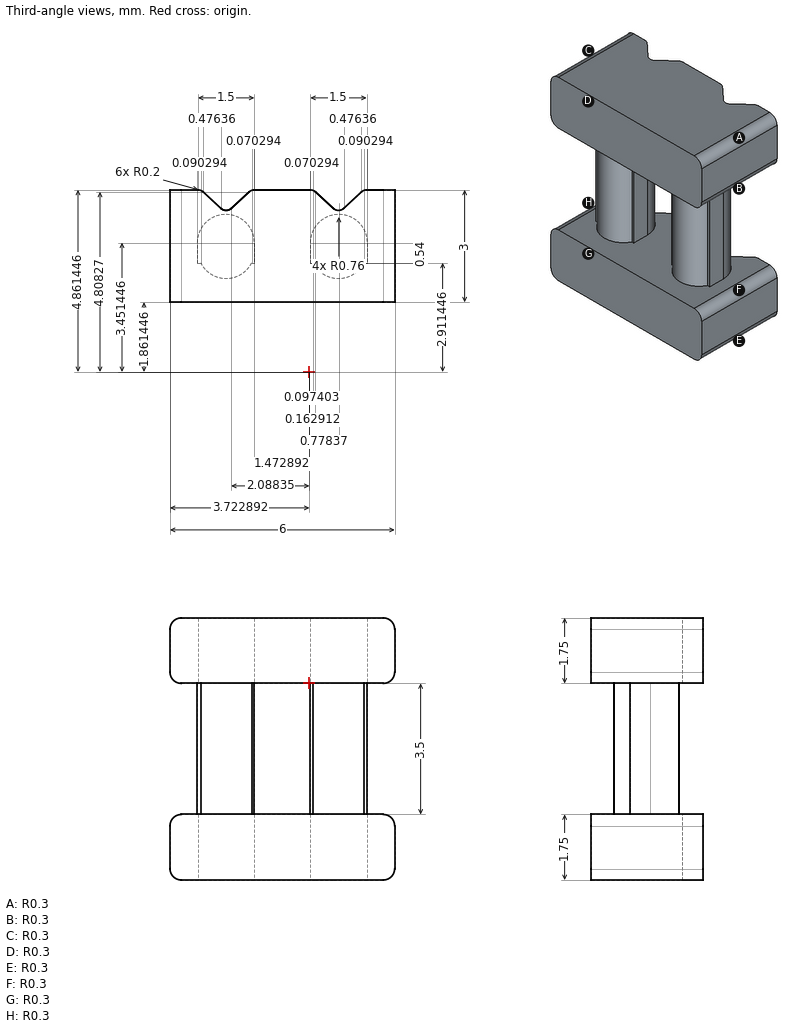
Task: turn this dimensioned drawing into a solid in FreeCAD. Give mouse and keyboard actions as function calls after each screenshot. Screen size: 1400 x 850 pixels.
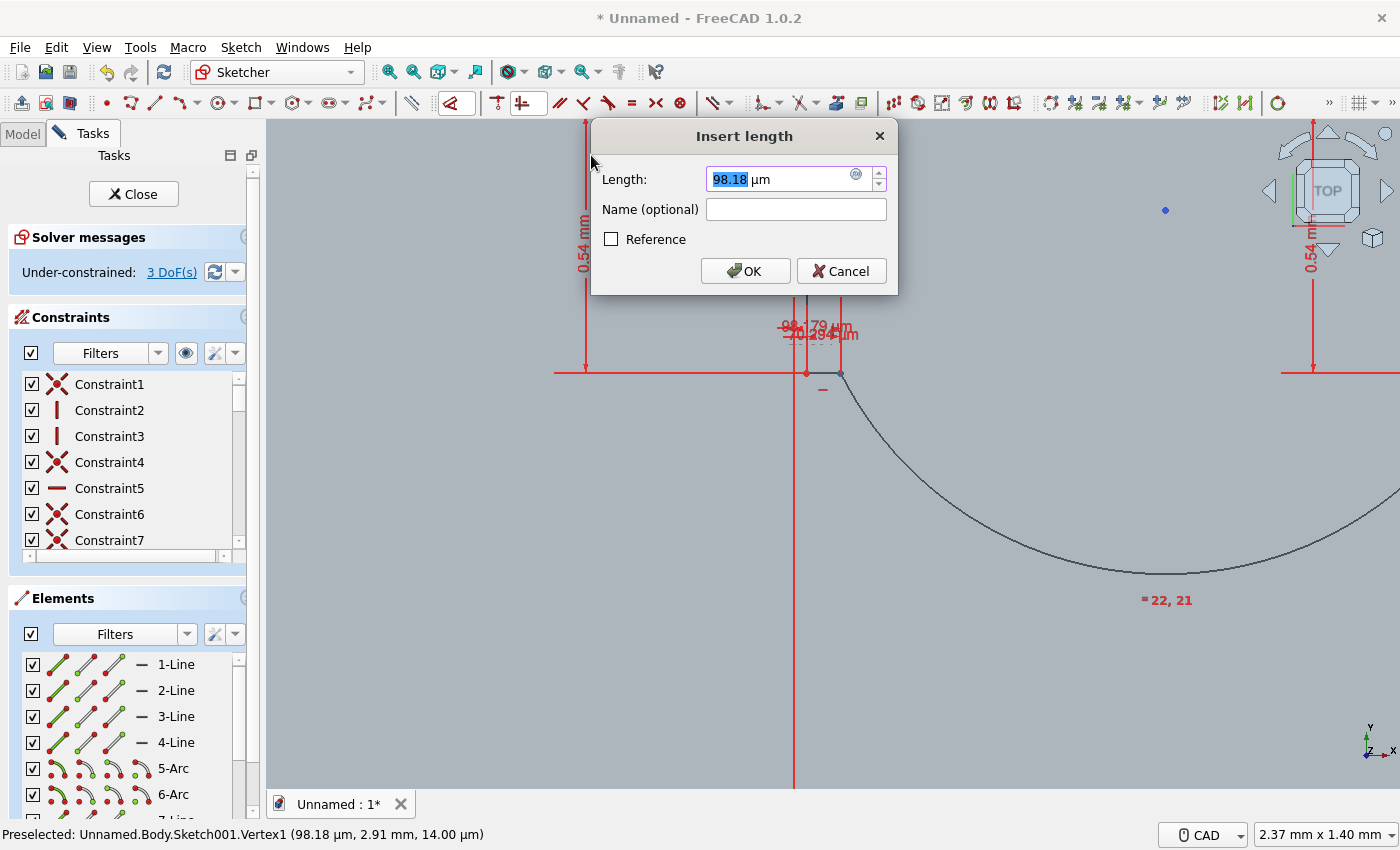
key(ctrl+a)
text(0.097403 mm)
key(Return)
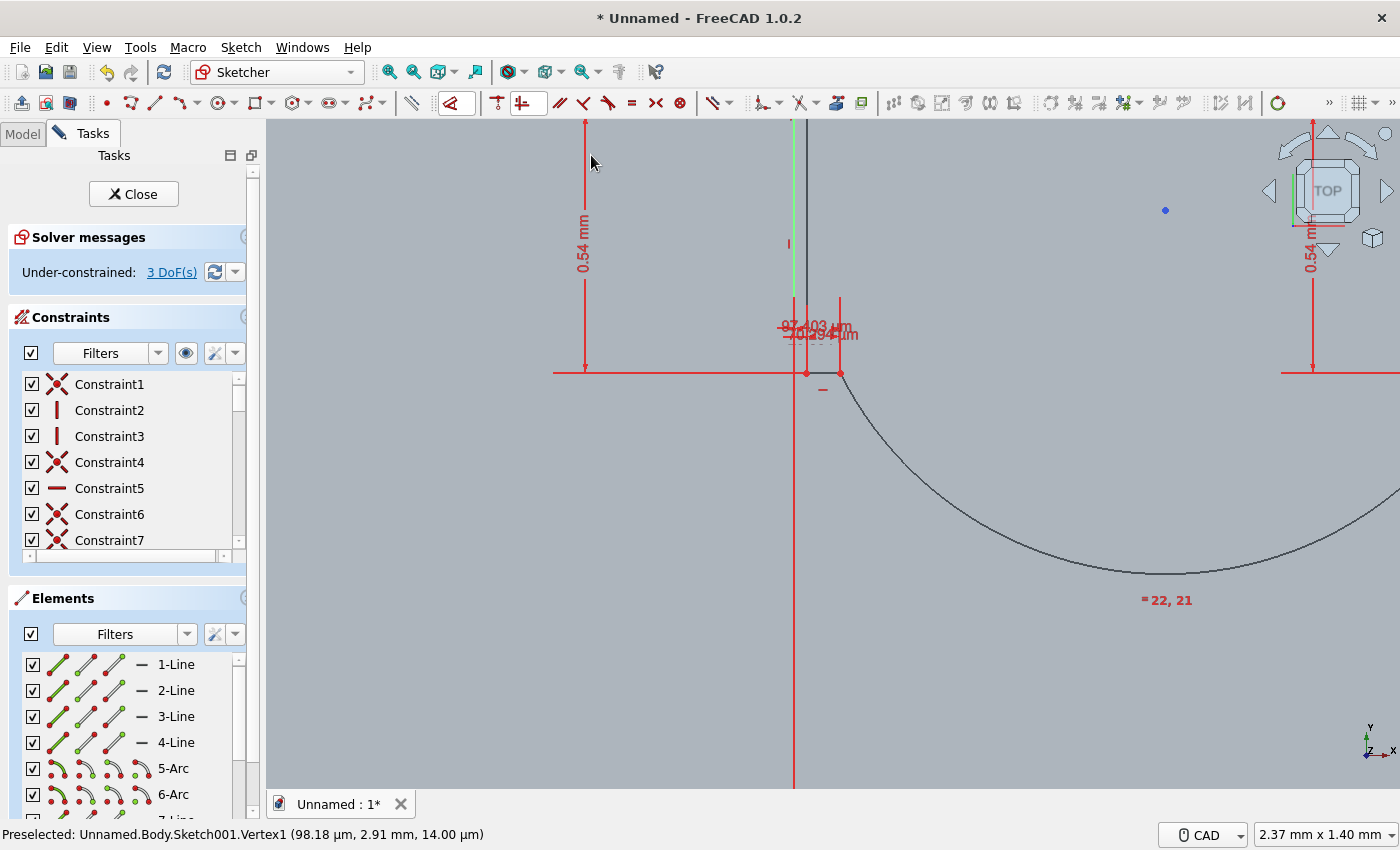
click(840, 373)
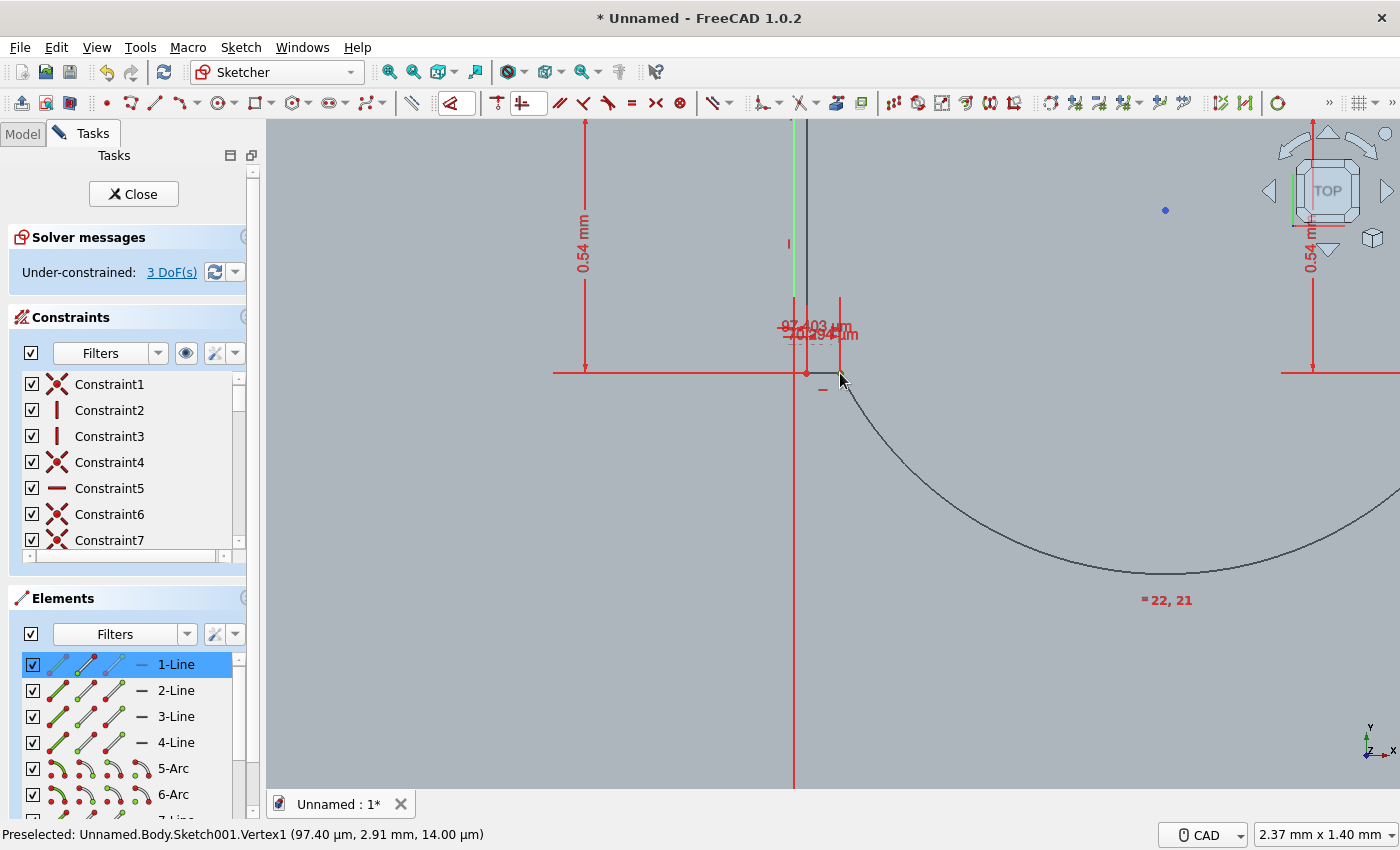
key(i)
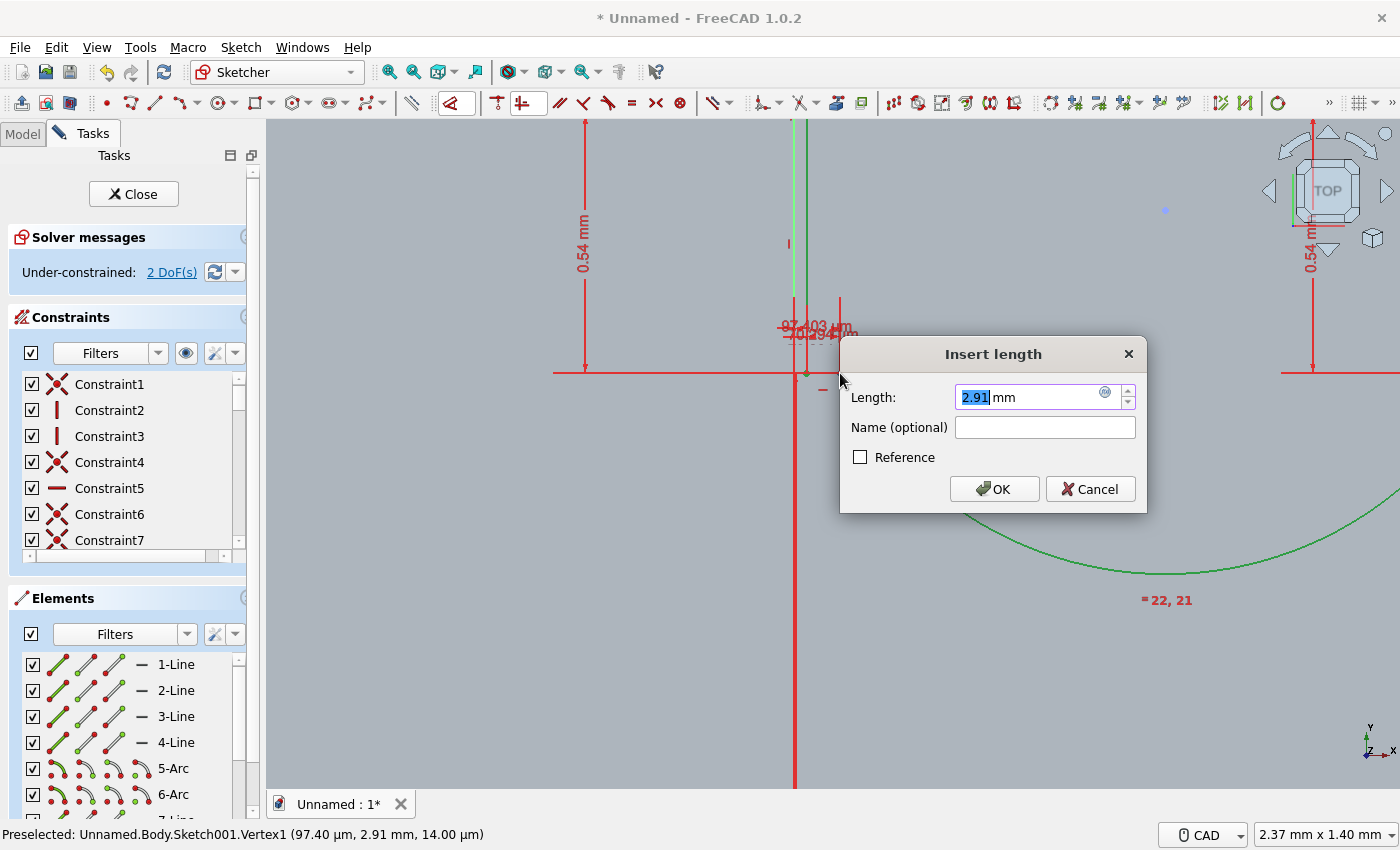
text(2.911446)
key(Return)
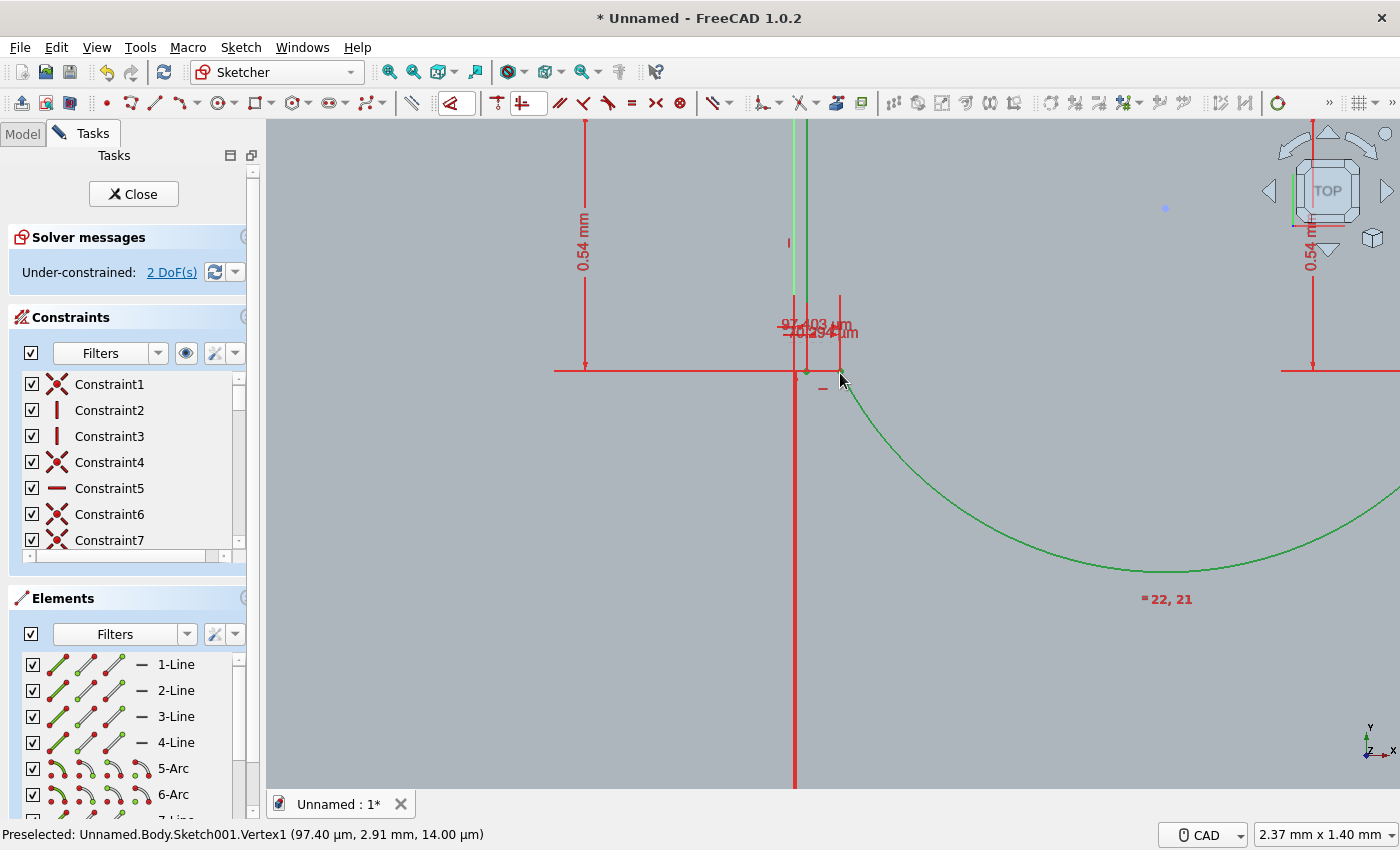
scroll(845, 377, down, 8)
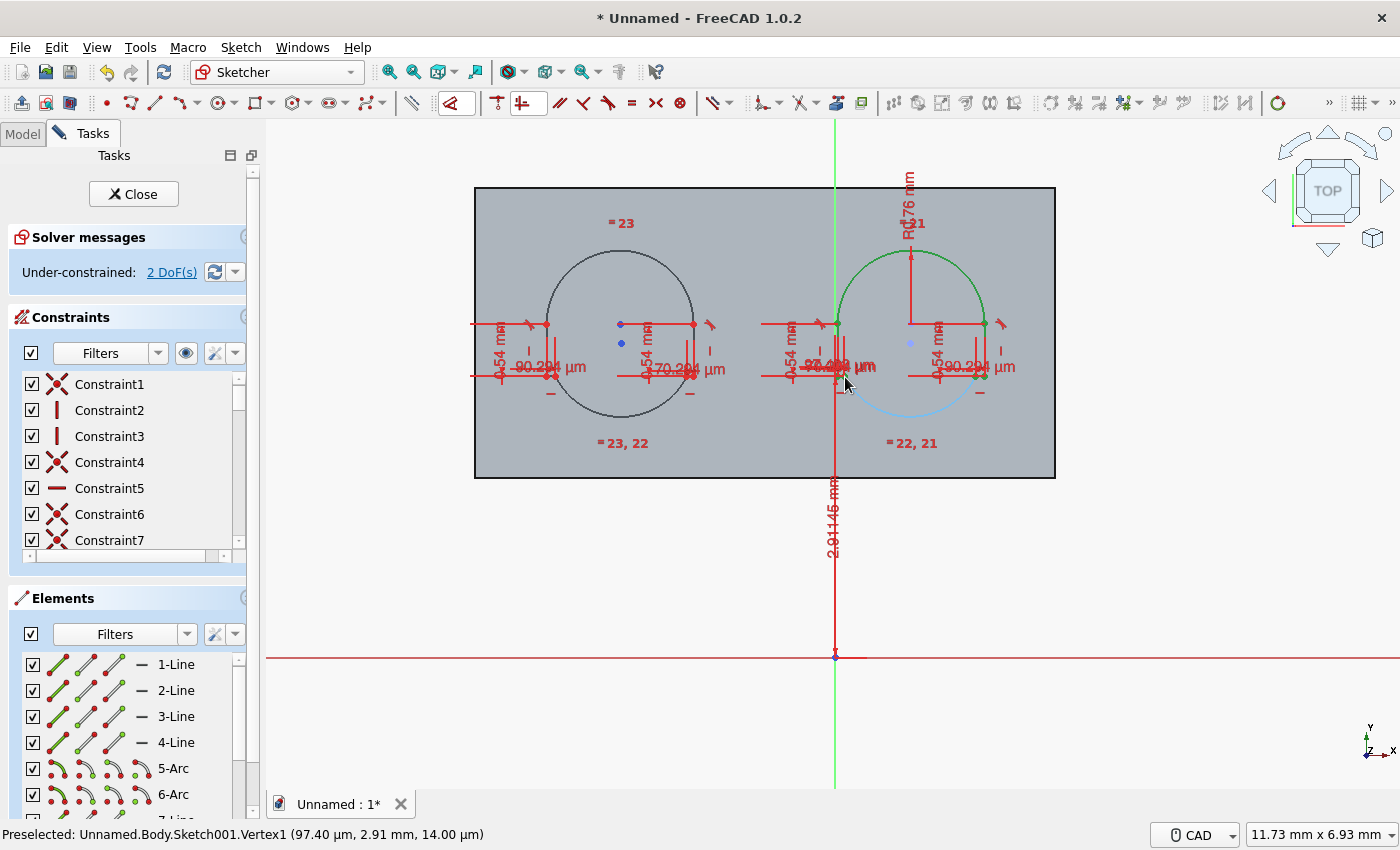
click(694, 324)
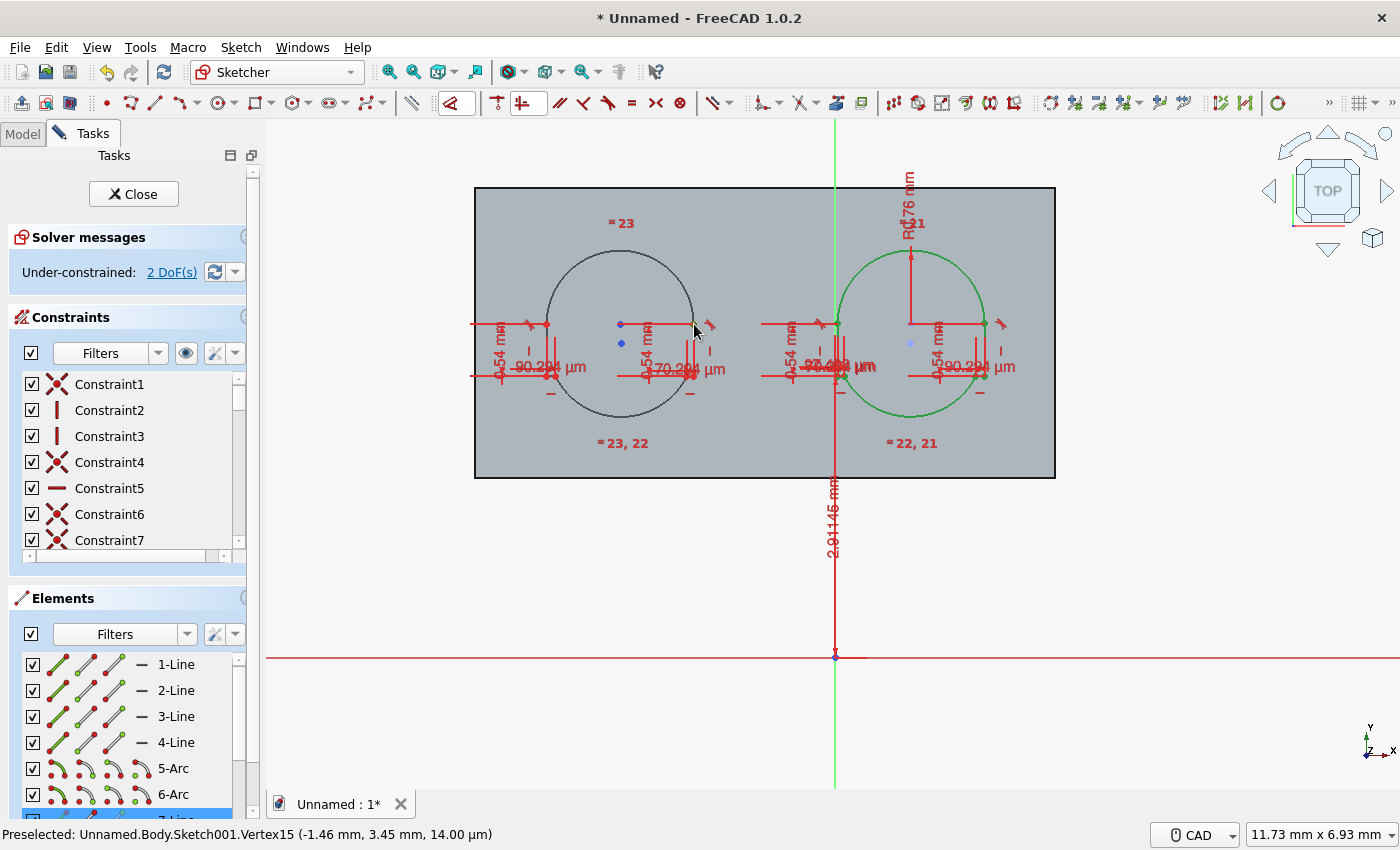
key(l)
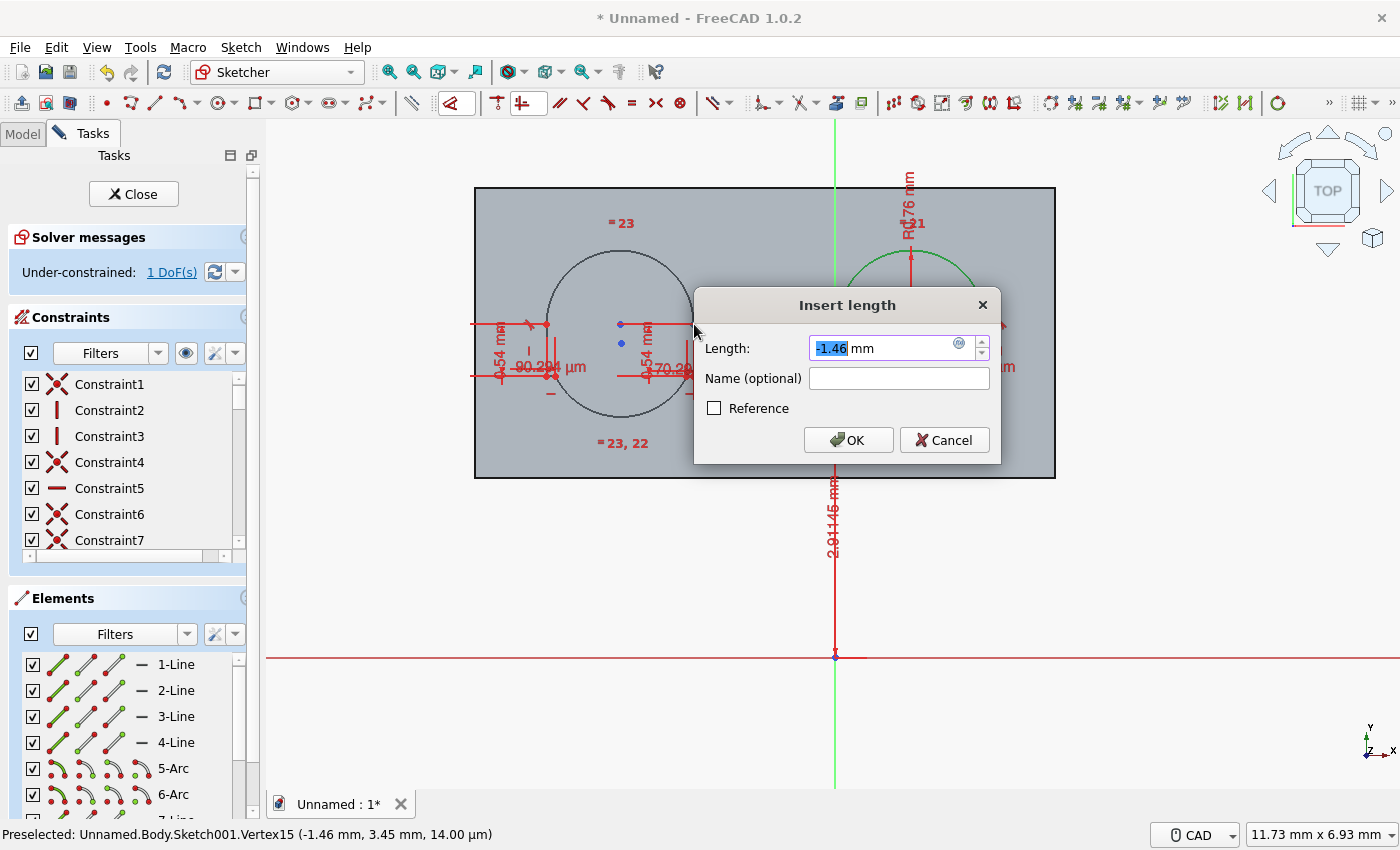
text(-1.472892)
key(Return)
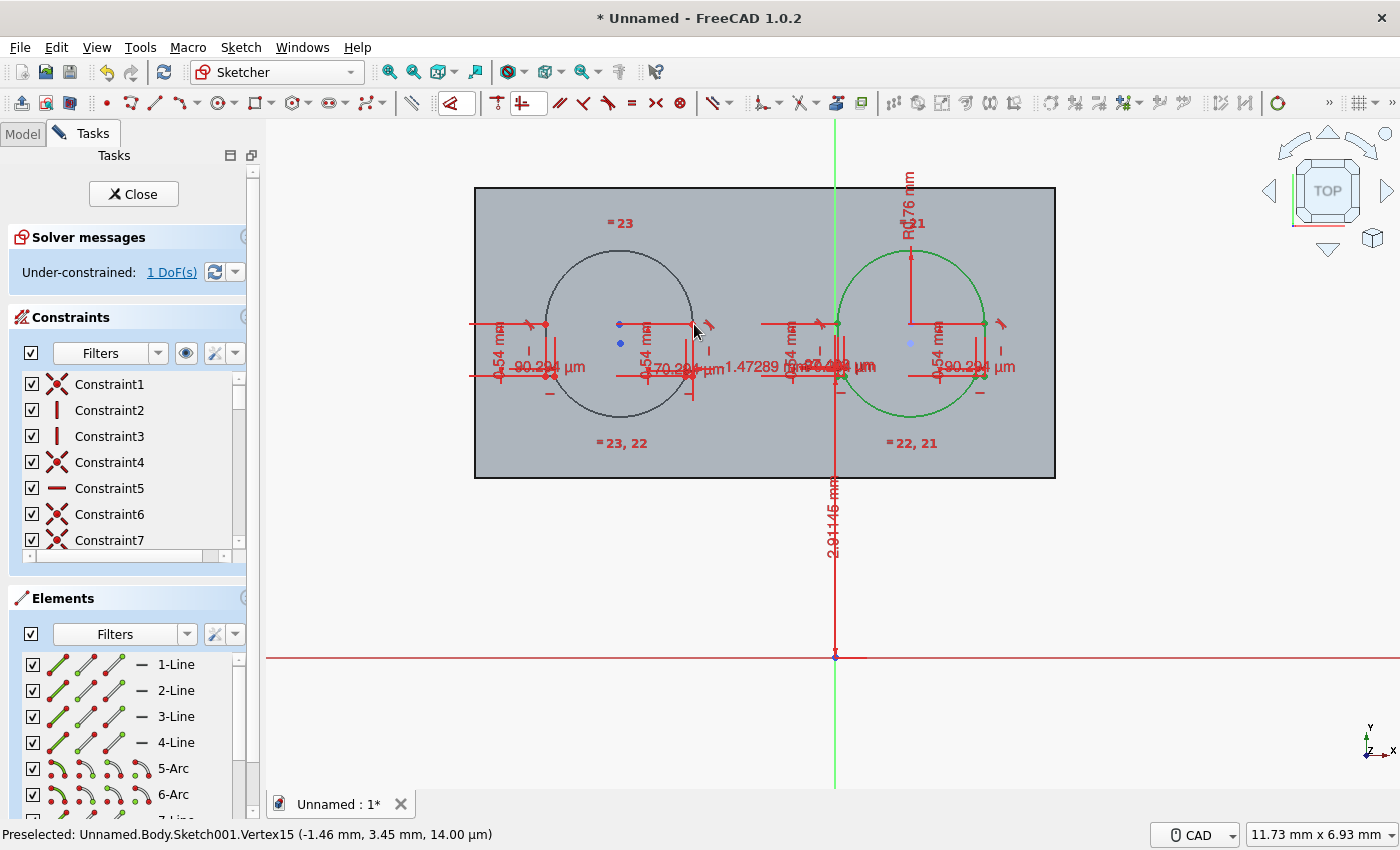
click(693, 324)